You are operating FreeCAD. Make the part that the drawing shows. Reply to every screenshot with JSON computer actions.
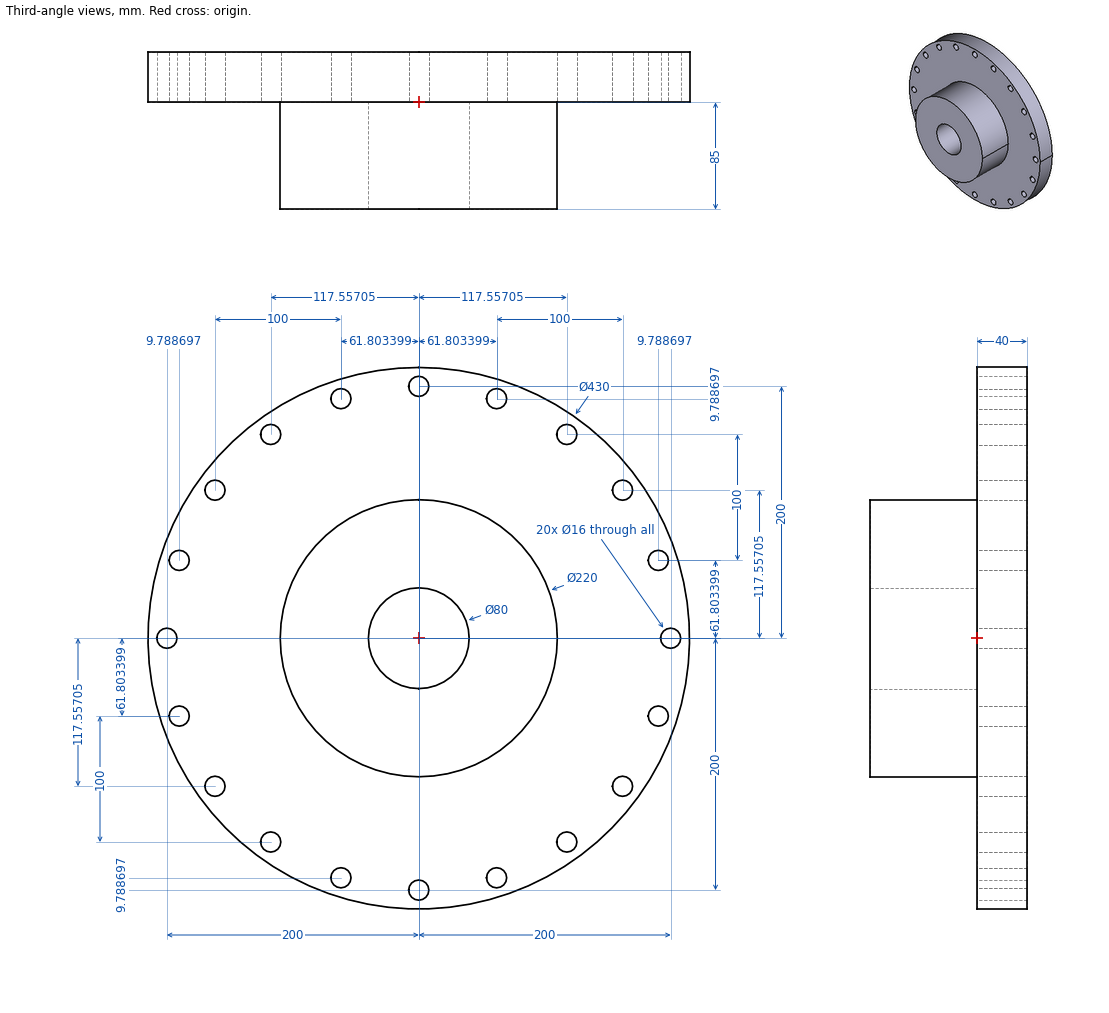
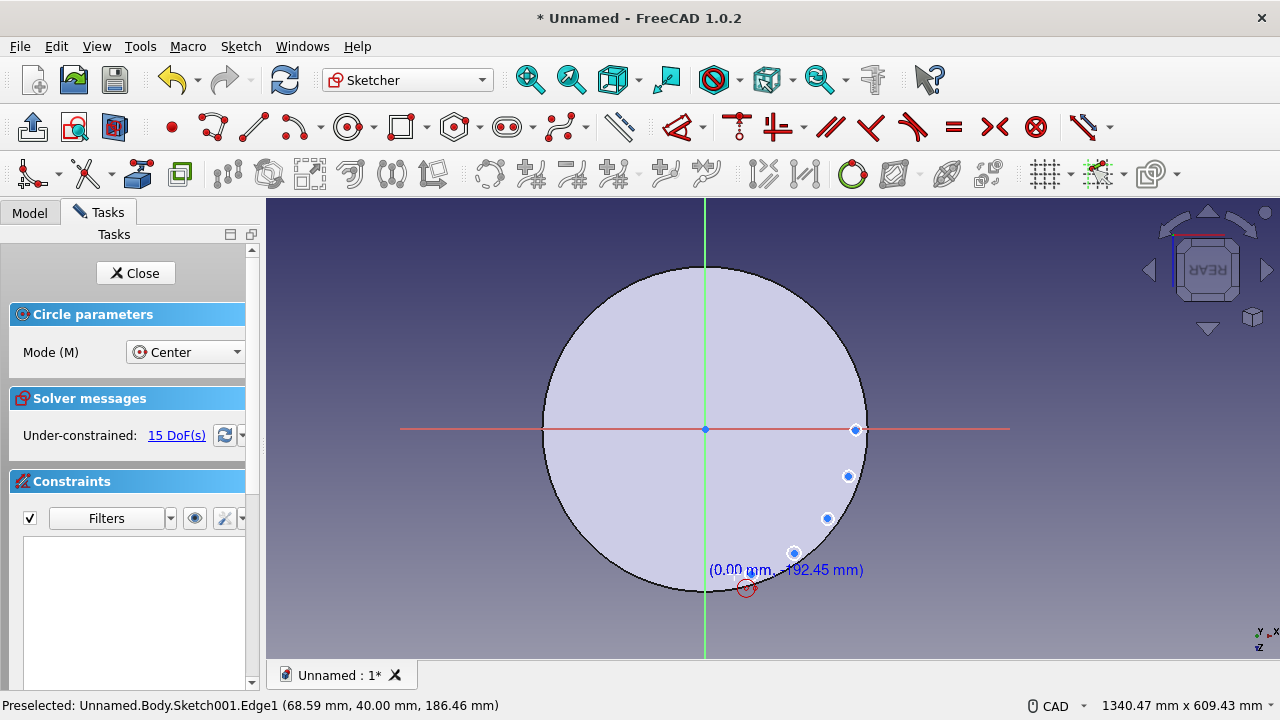
{"action": "left_click", "coordinate": [705, 581]}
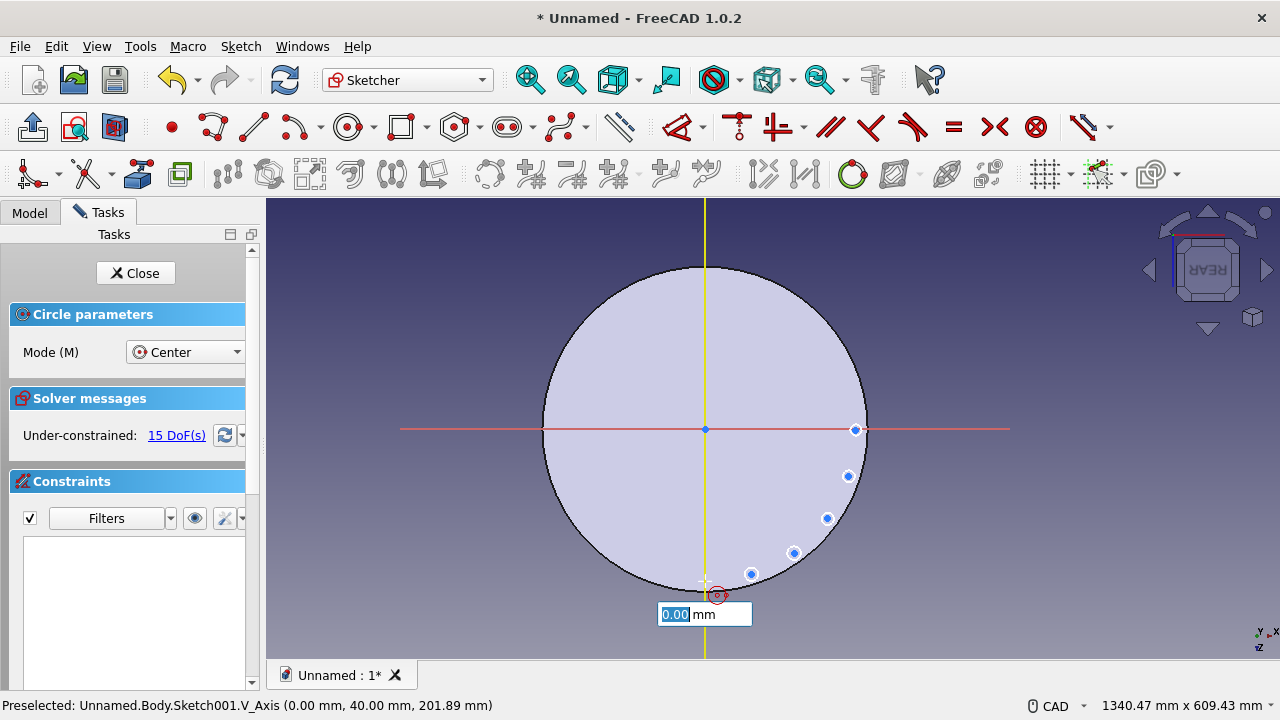
{"action": "scroll", "coordinate": [711, 579], "scroll_direction": "up", "scroll_amount": 6}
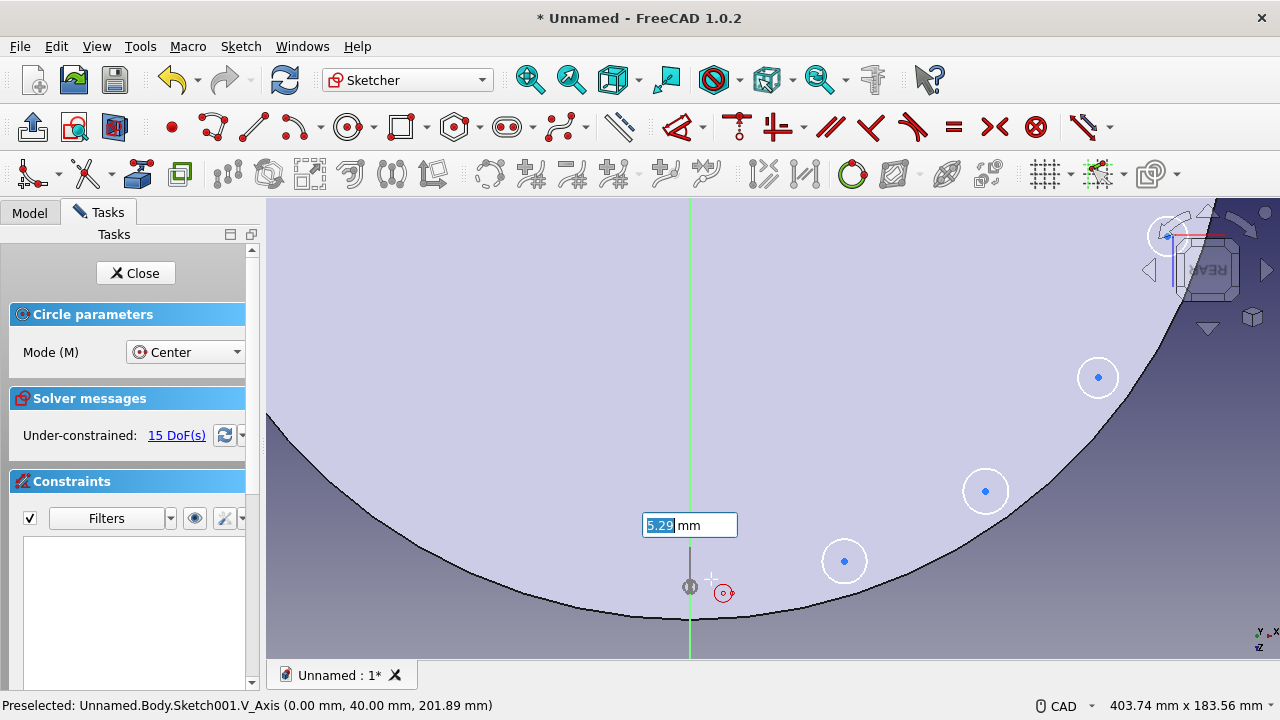
{"action": "left_click", "coordinate": [709, 575]}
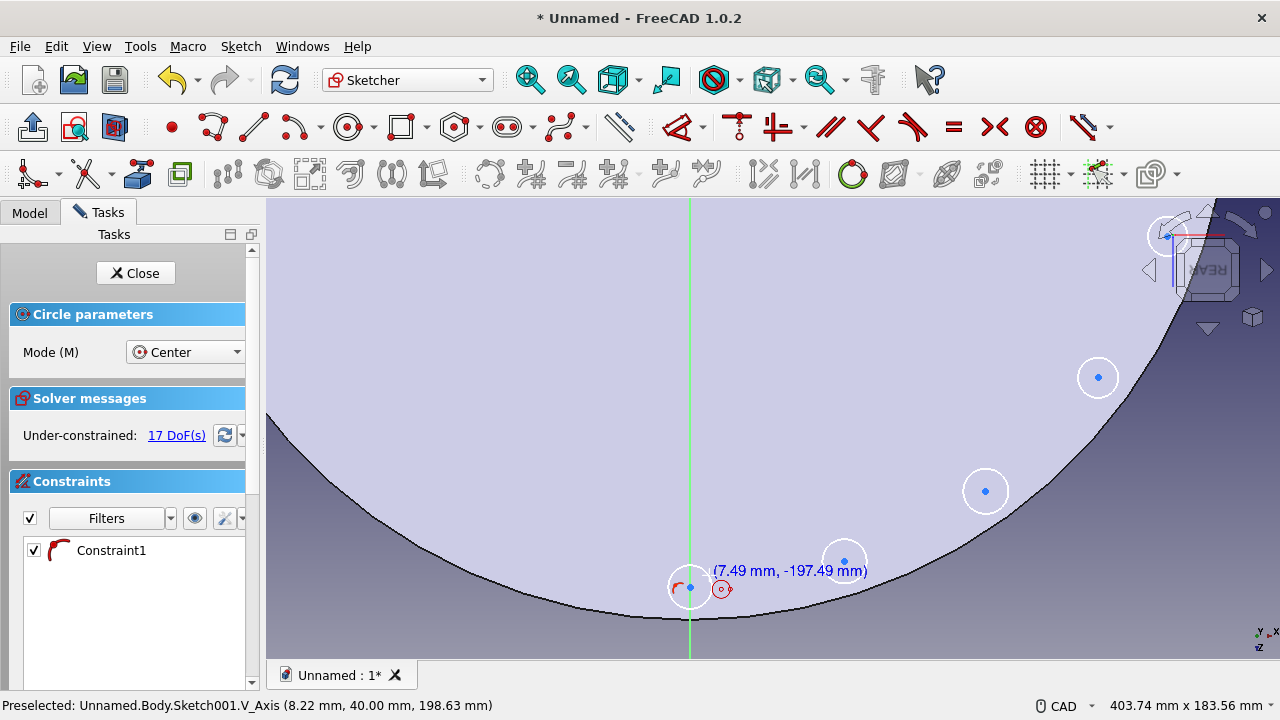
{"action": "left_click", "coordinate": [535, 558]}
{"action": "left_click", "coordinate": [549, 544]}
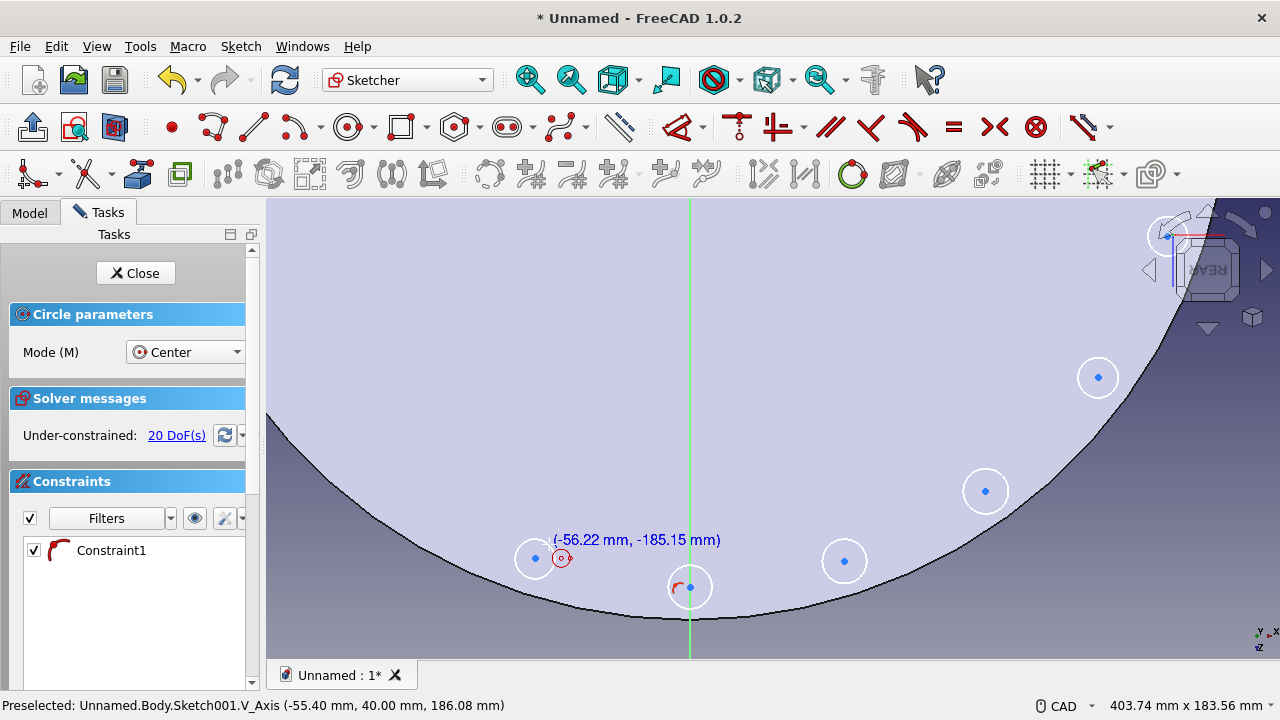
{"action": "left_click", "coordinate": [395, 486]}
{"action": "left_click", "coordinate": [409, 472]}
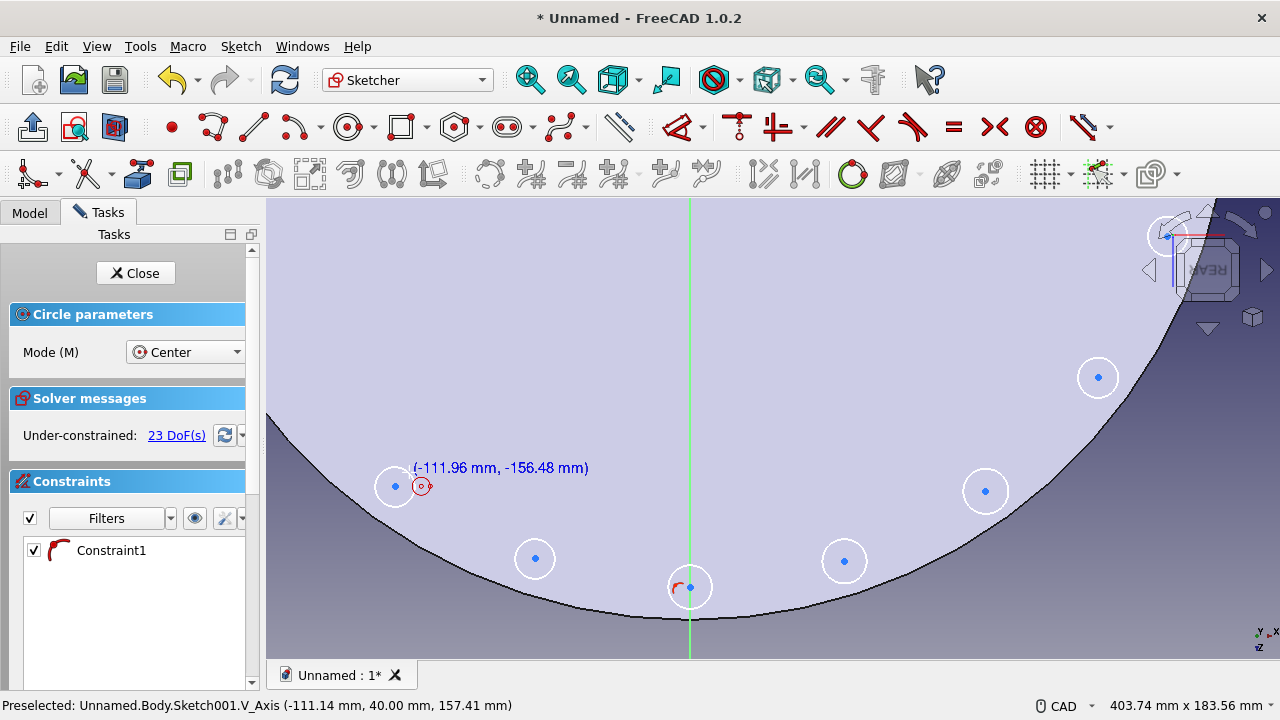
{"action": "scroll", "coordinate": [711, 579], "scroll_direction": "down", "scroll_amount": 6}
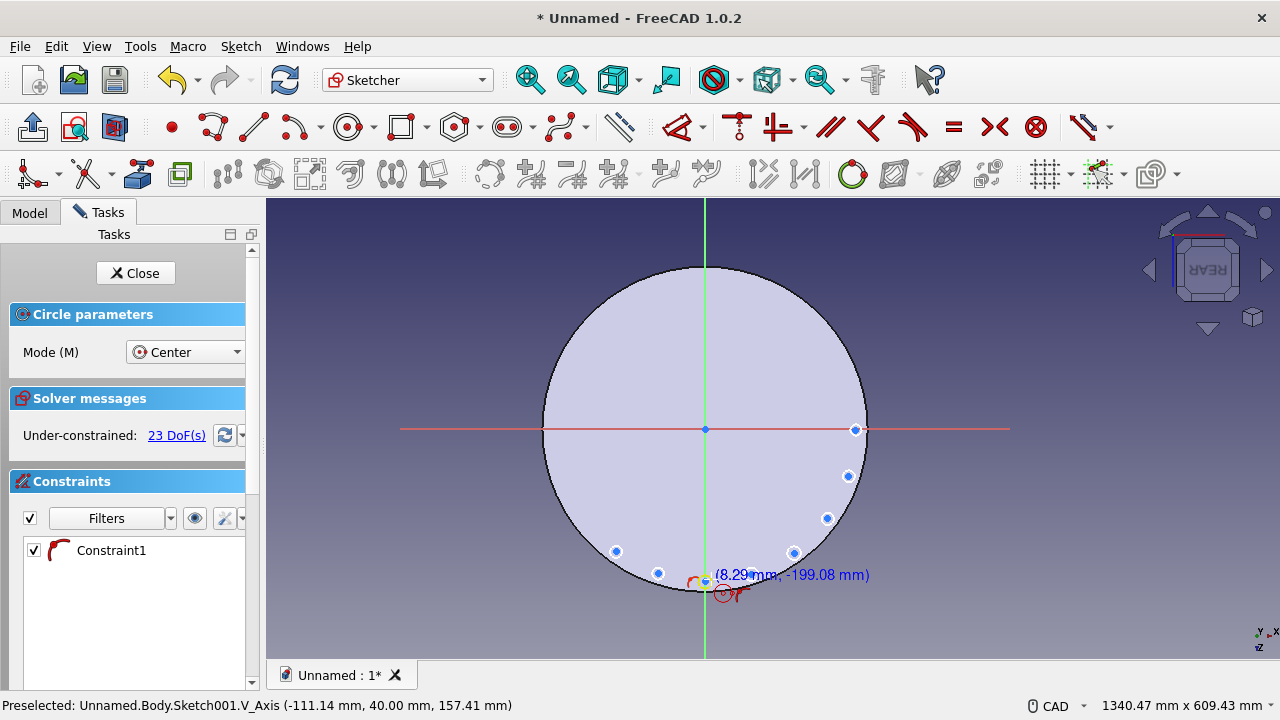
{"action": "scroll", "coordinate": [583, 518], "scroll_direction": "up", "scroll_amount": 7}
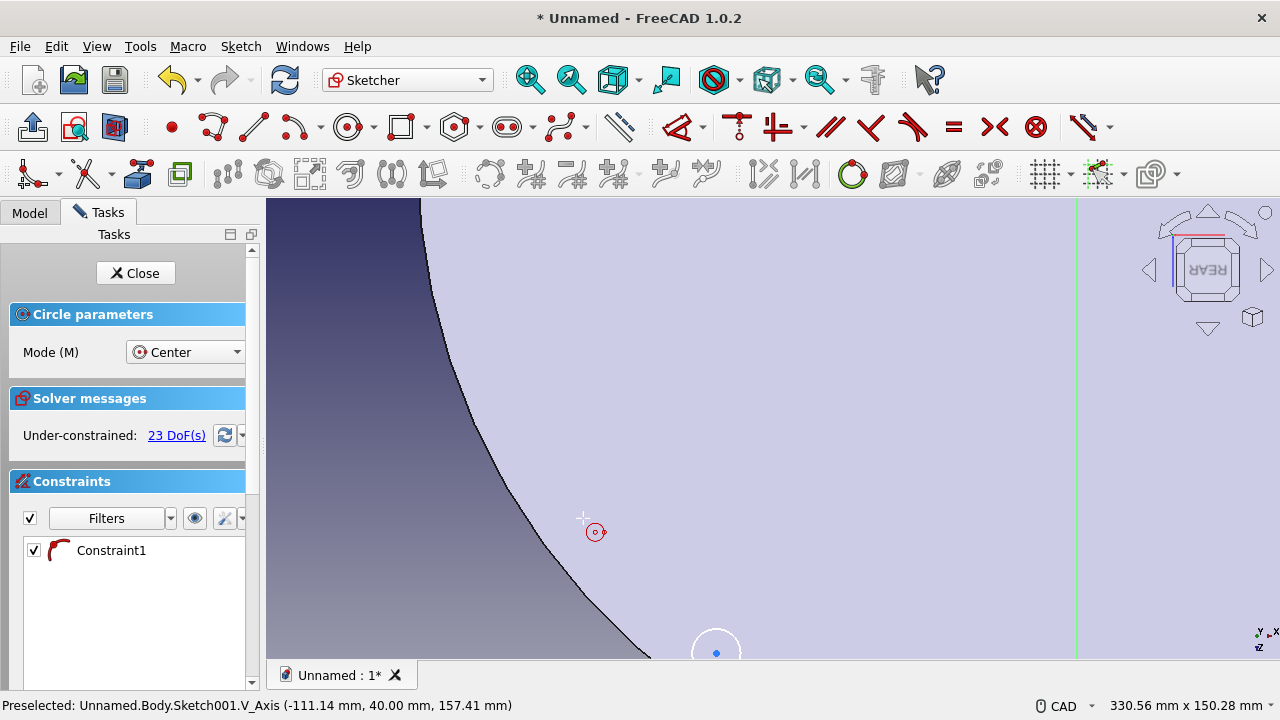
{"action": "scroll", "coordinate": [583, 518], "scroll_direction": "down", "scroll_amount": 7}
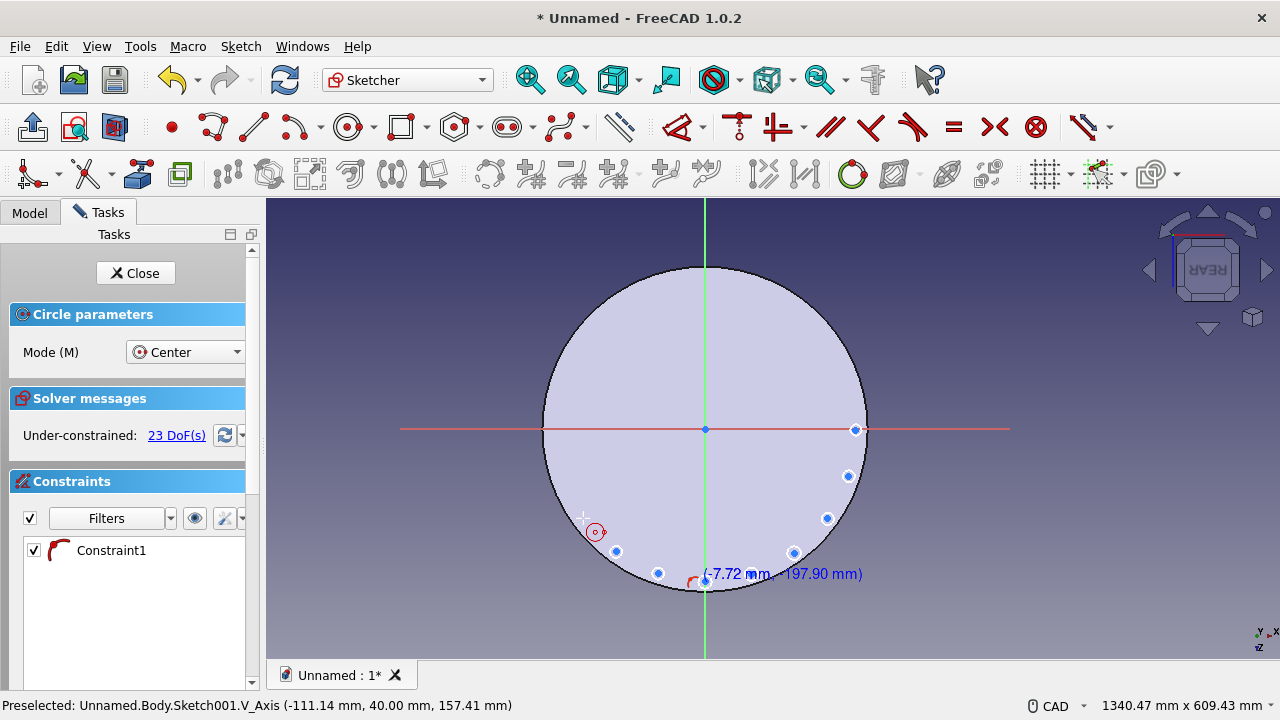
{"action": "left_click", "coordinate": [583, 518]}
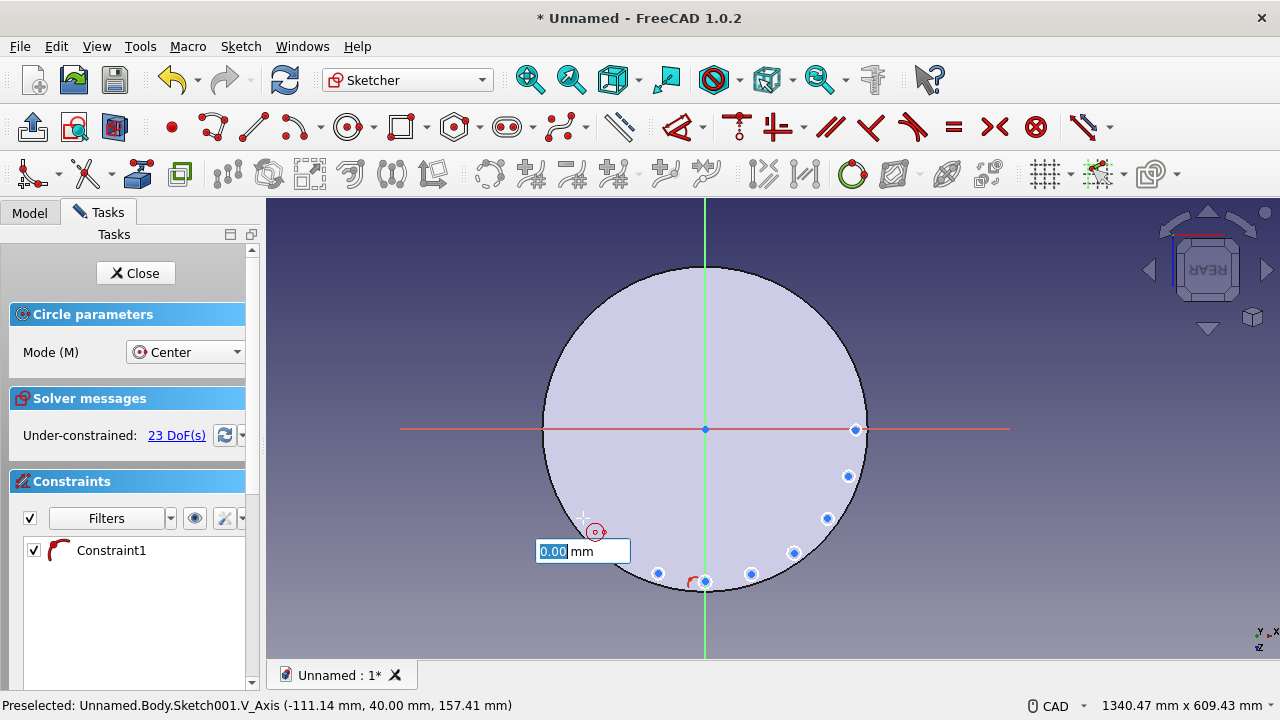
{"action": "scroll", "coordinate": [587, 514], "scroll_direction": "up", "scroll_amount": 5}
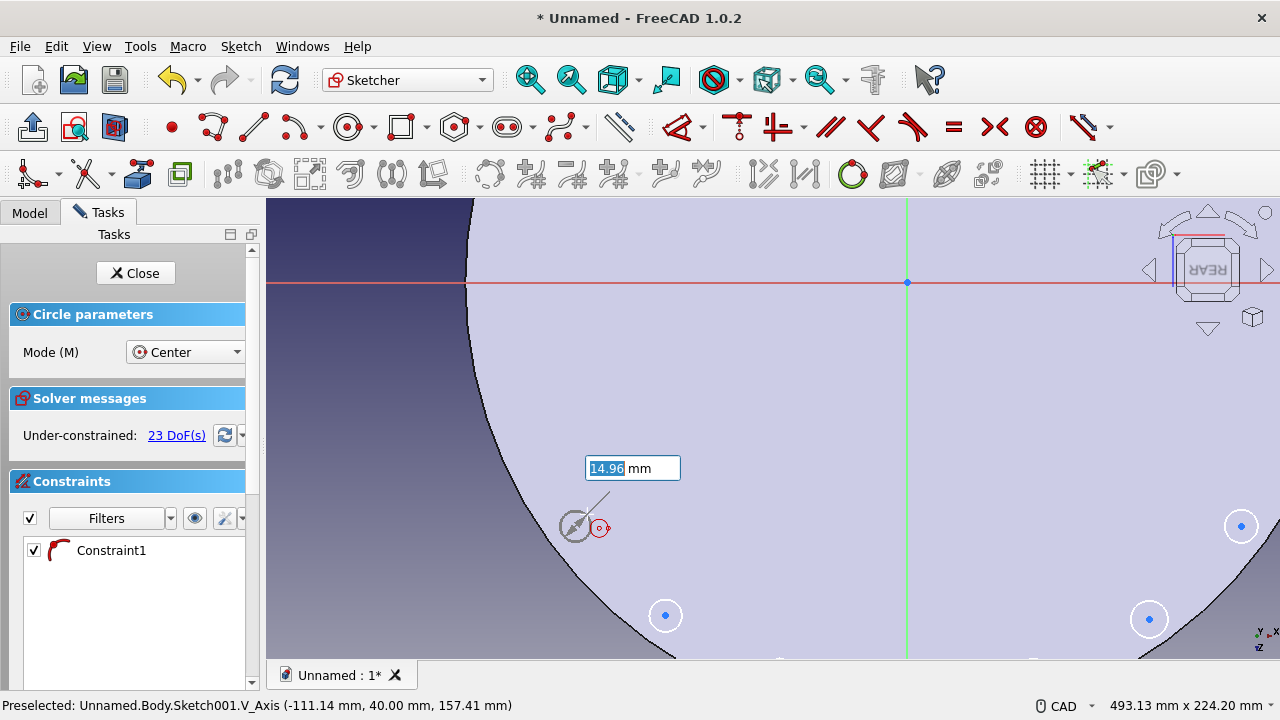
{"action": "left_click", "coordinate": [586, 513]}